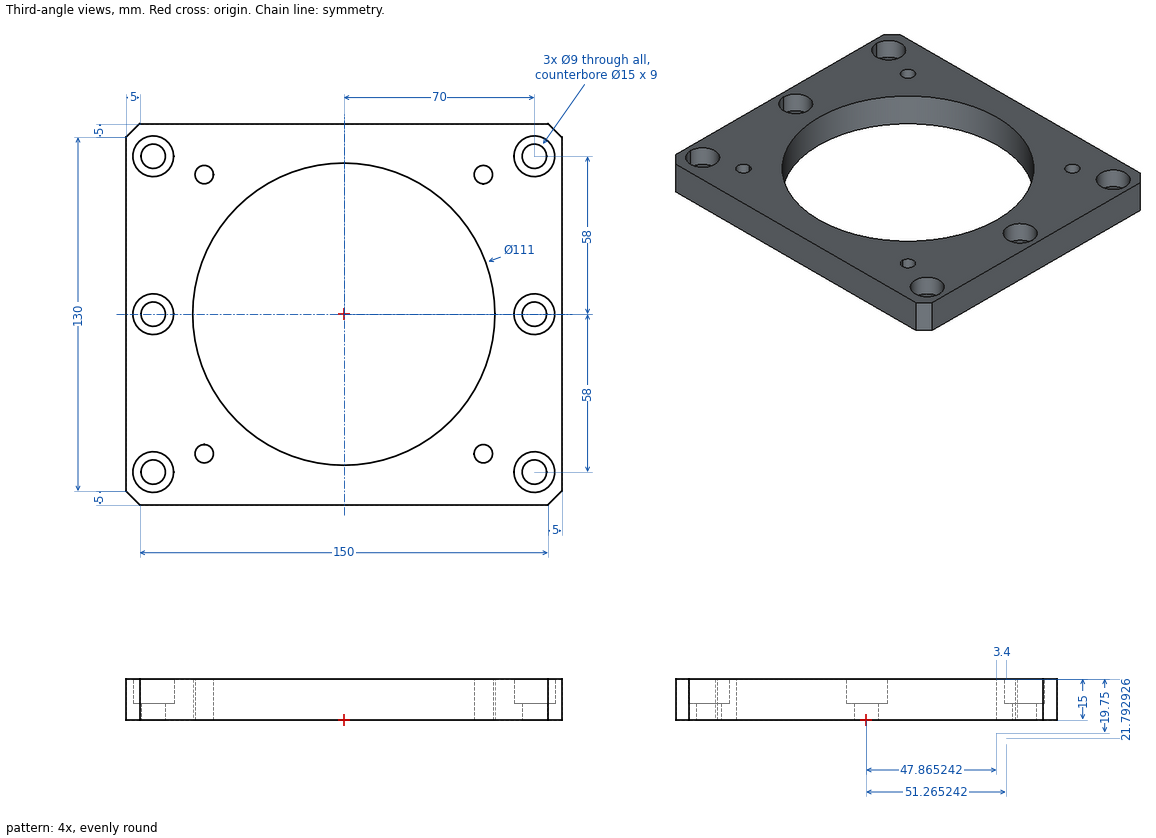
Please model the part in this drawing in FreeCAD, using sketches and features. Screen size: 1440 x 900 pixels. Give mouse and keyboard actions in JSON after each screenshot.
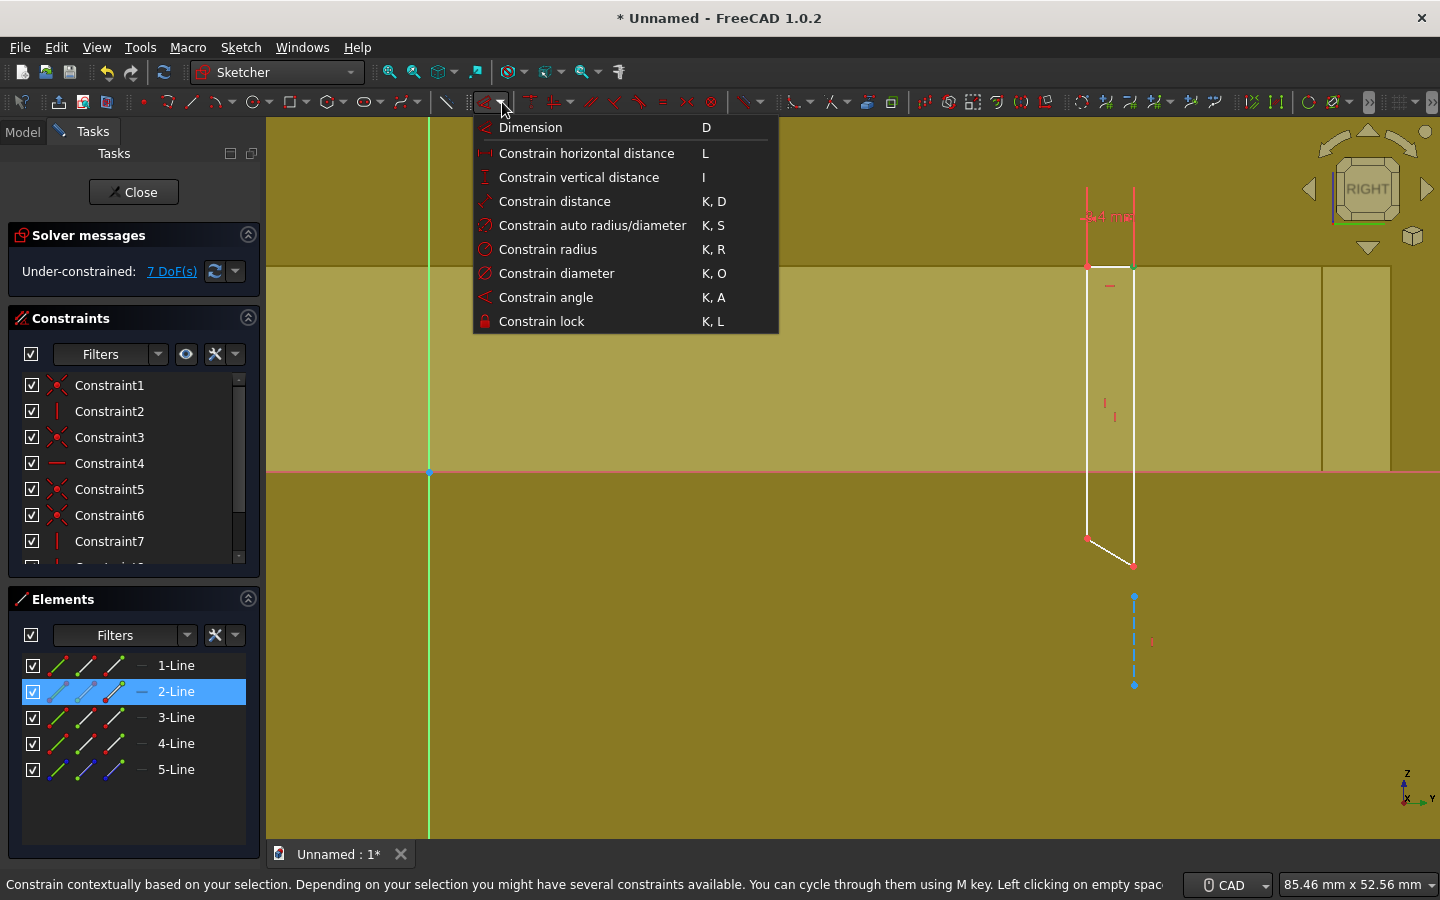
{"action": "left_click", "coordinate": [626, 177]}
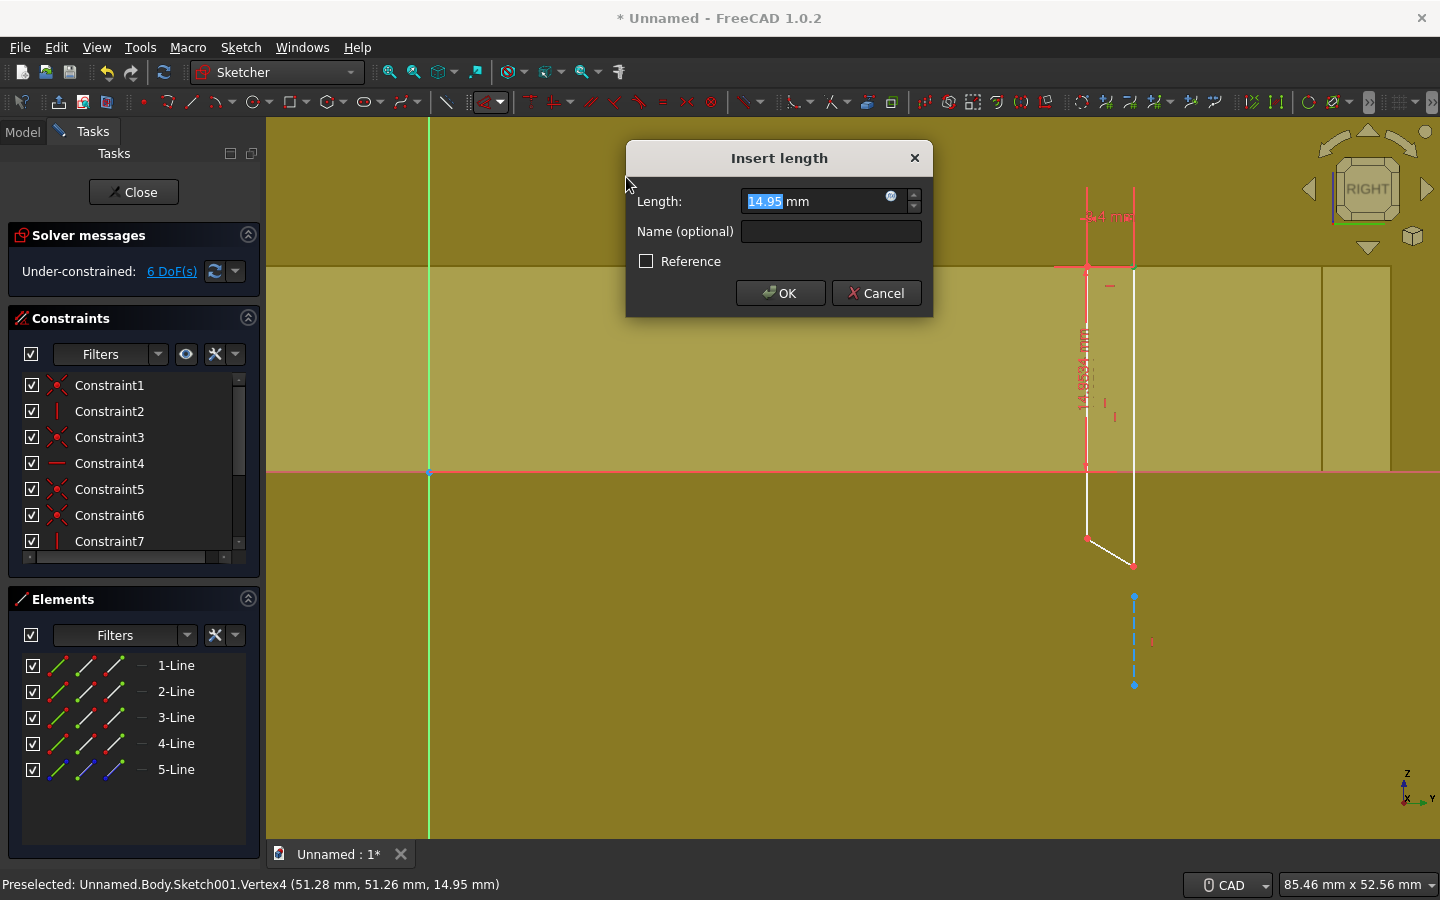
{"action": "type", "text": "15"}
{"action": "key", "text": "Return"}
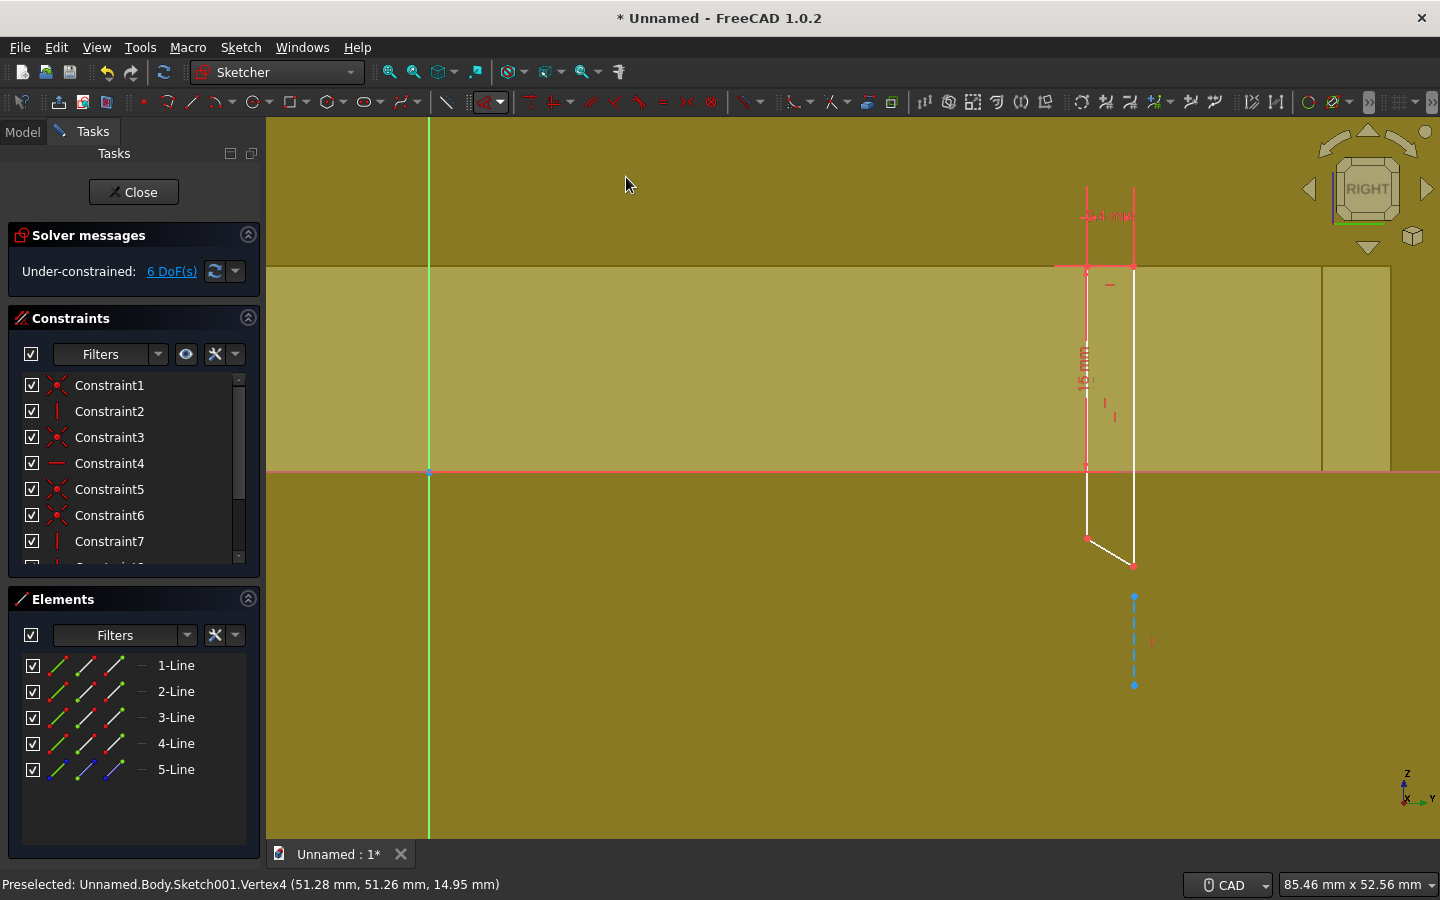
{"action": "left_click", "coordinate": [1087, 457]}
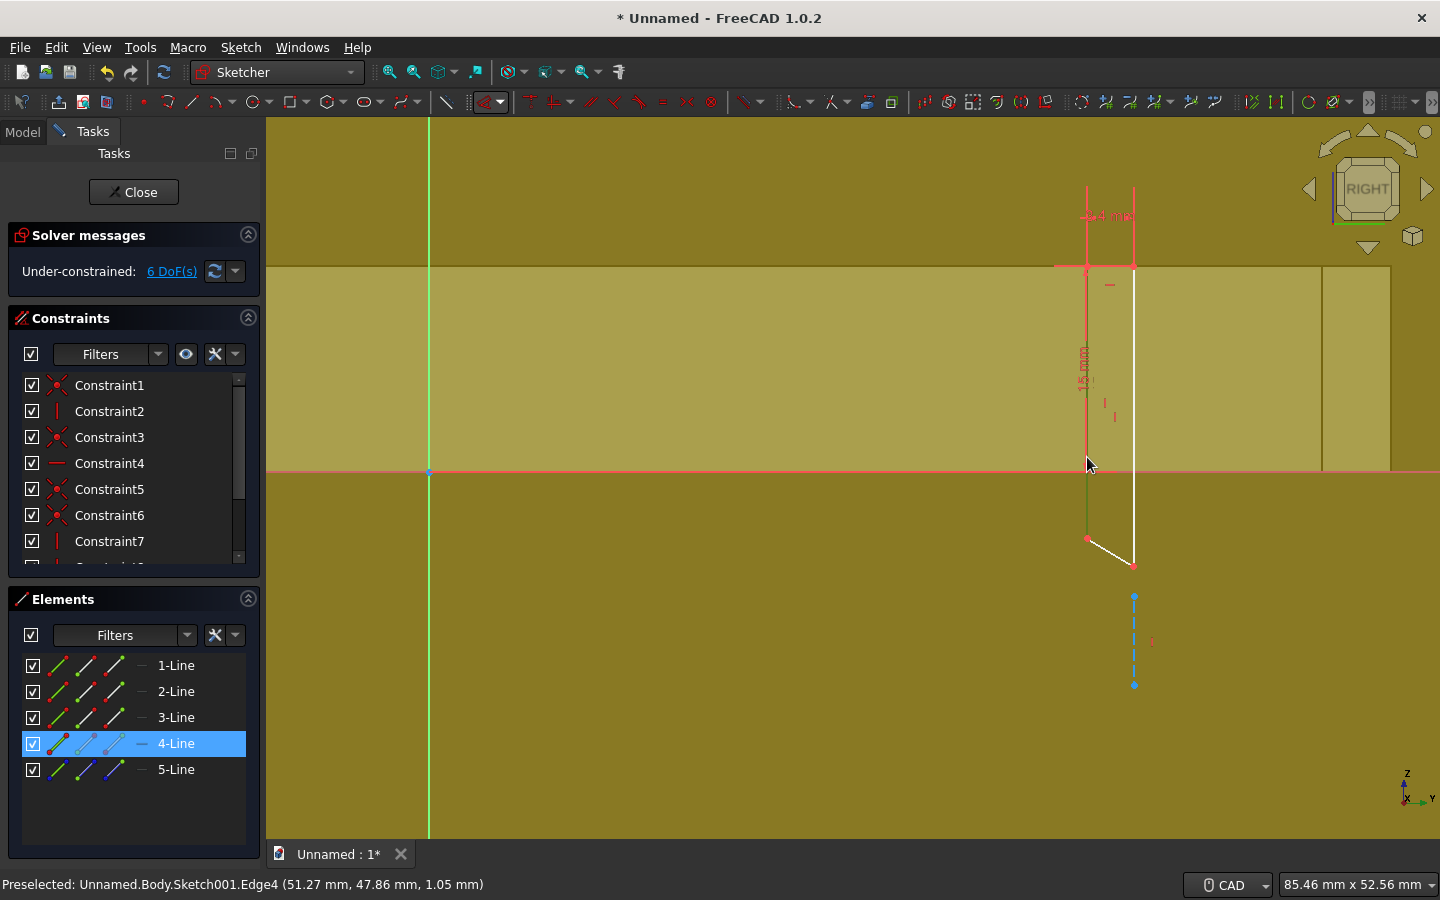
{"action": "key", "text": "i"}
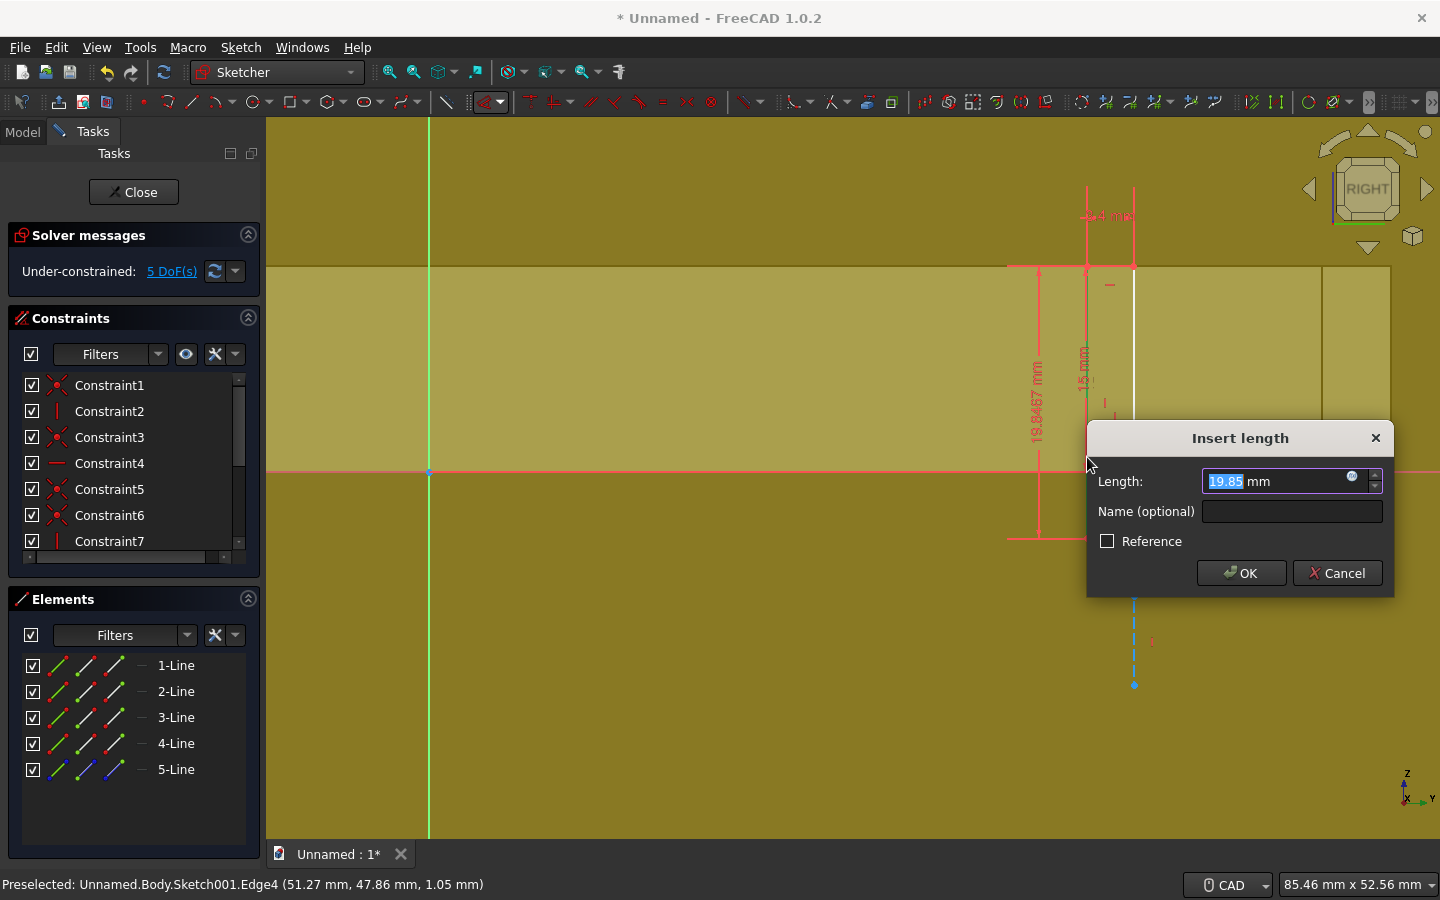
{"action": "type", "text": "19.75"}
{"action": "key", "text": "Return"}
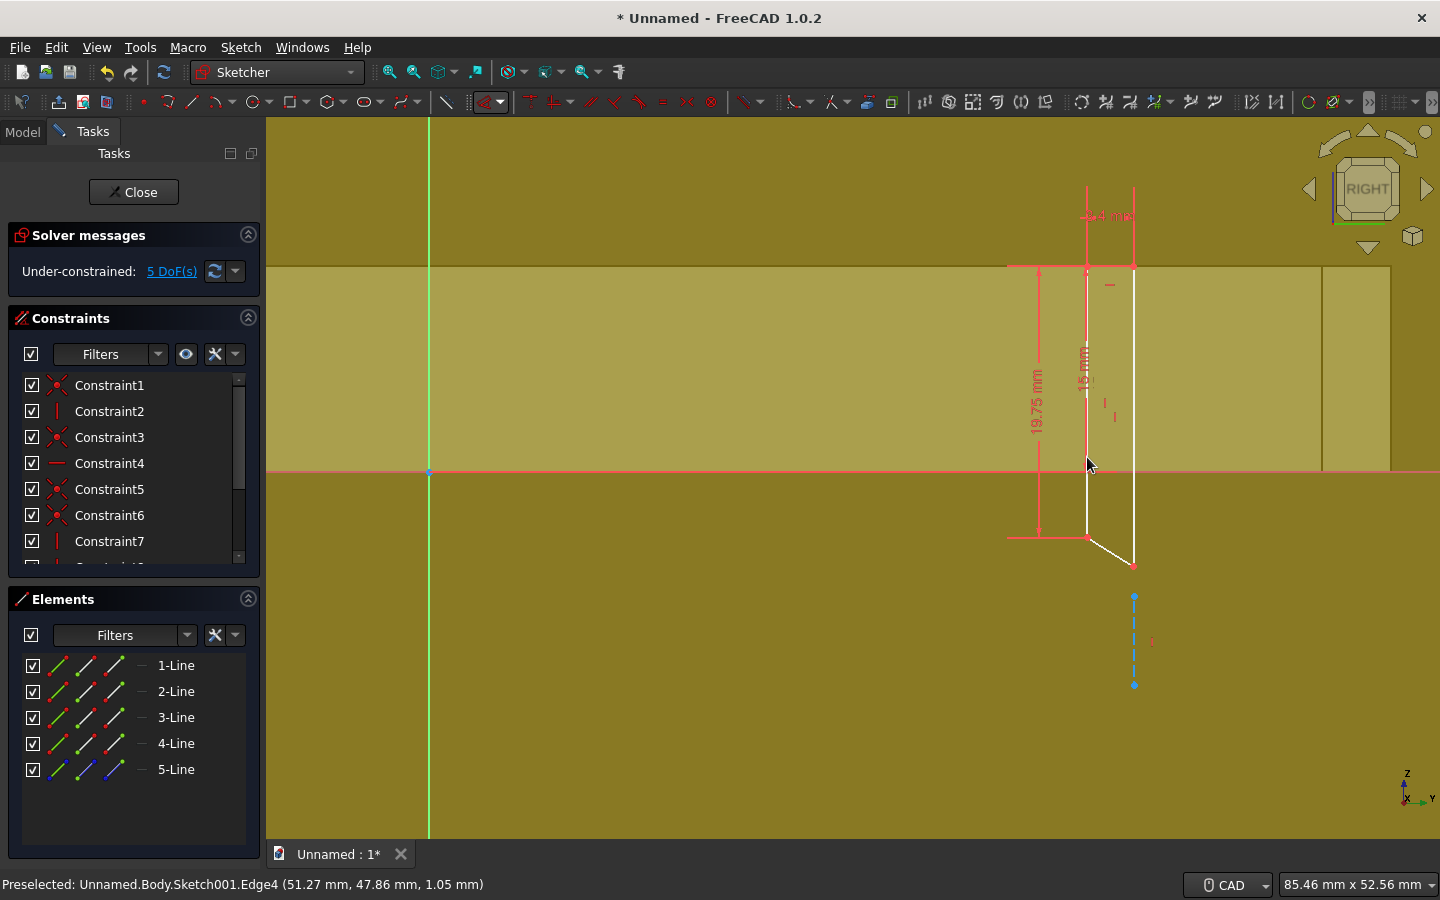
{"action": "left_click", "coordinate": [1134, 357]}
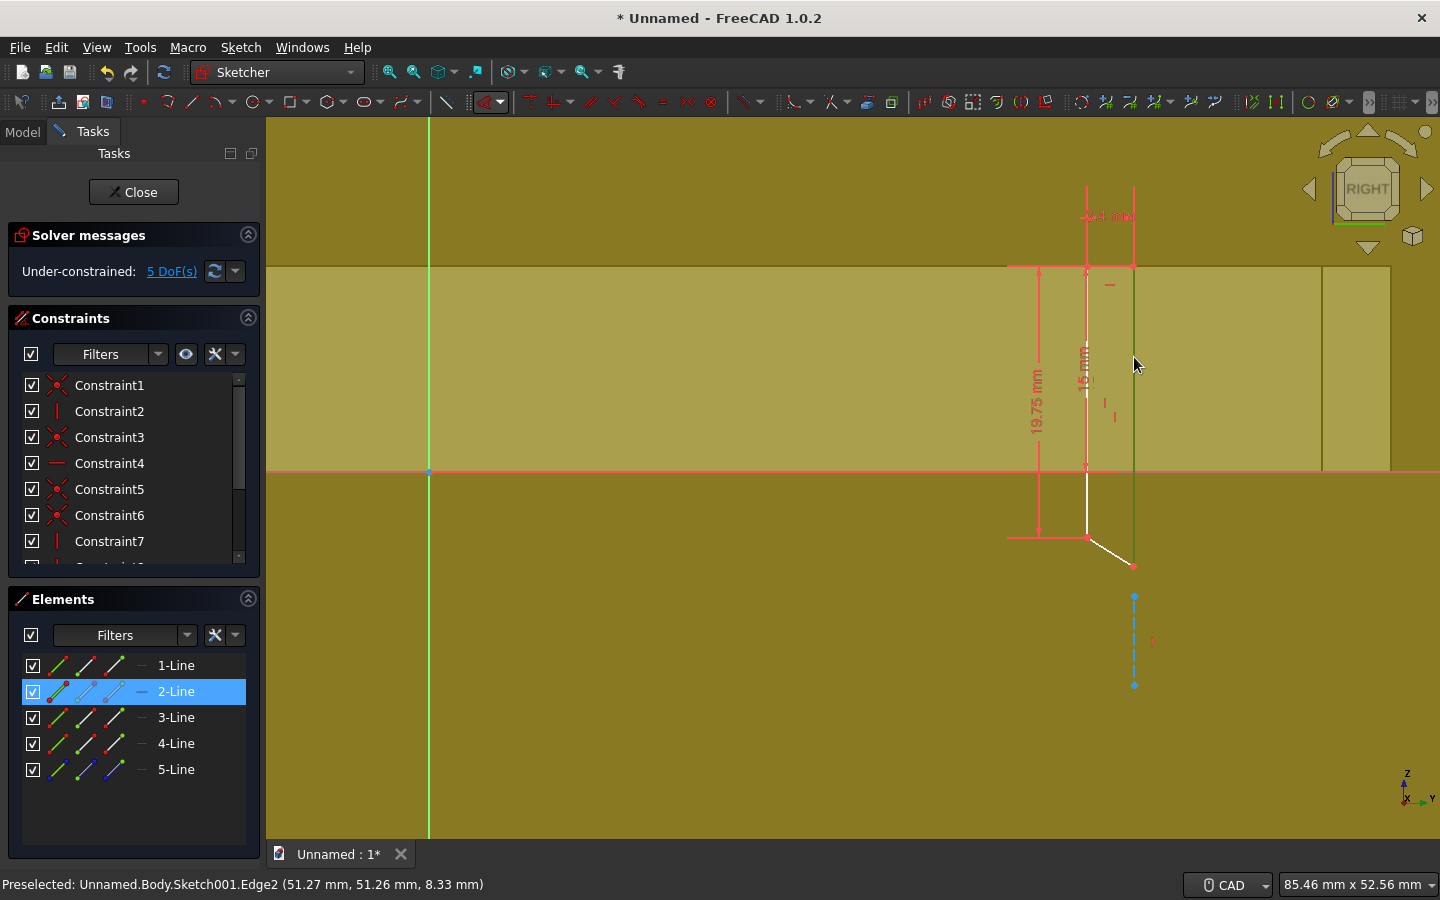
{"action": "left_click", "coordinate": [502, 102]}